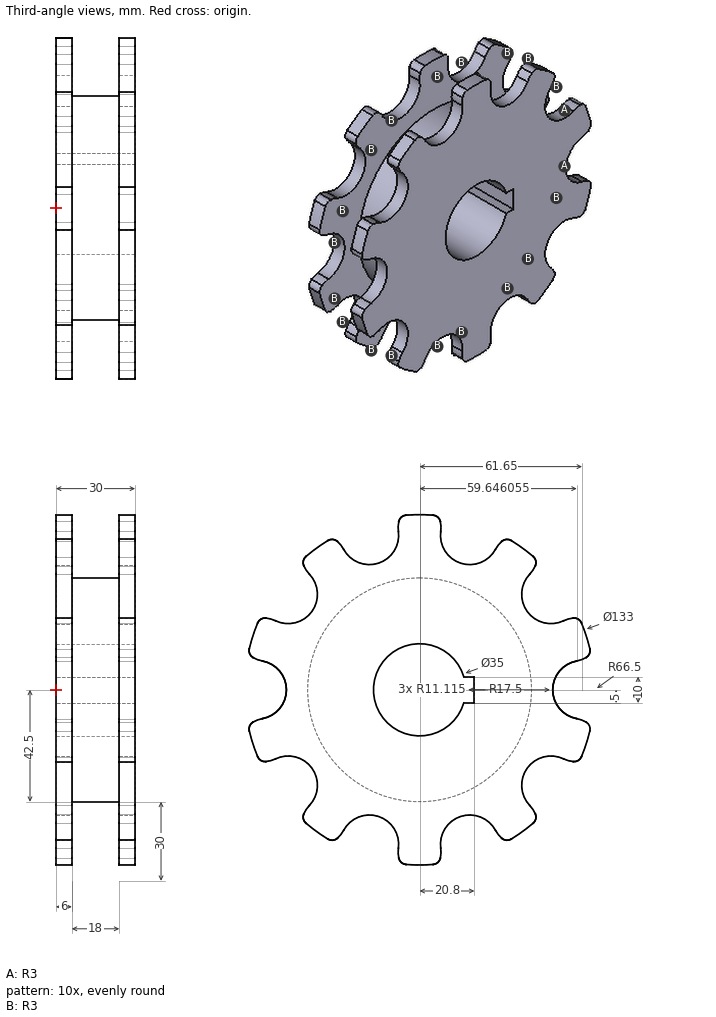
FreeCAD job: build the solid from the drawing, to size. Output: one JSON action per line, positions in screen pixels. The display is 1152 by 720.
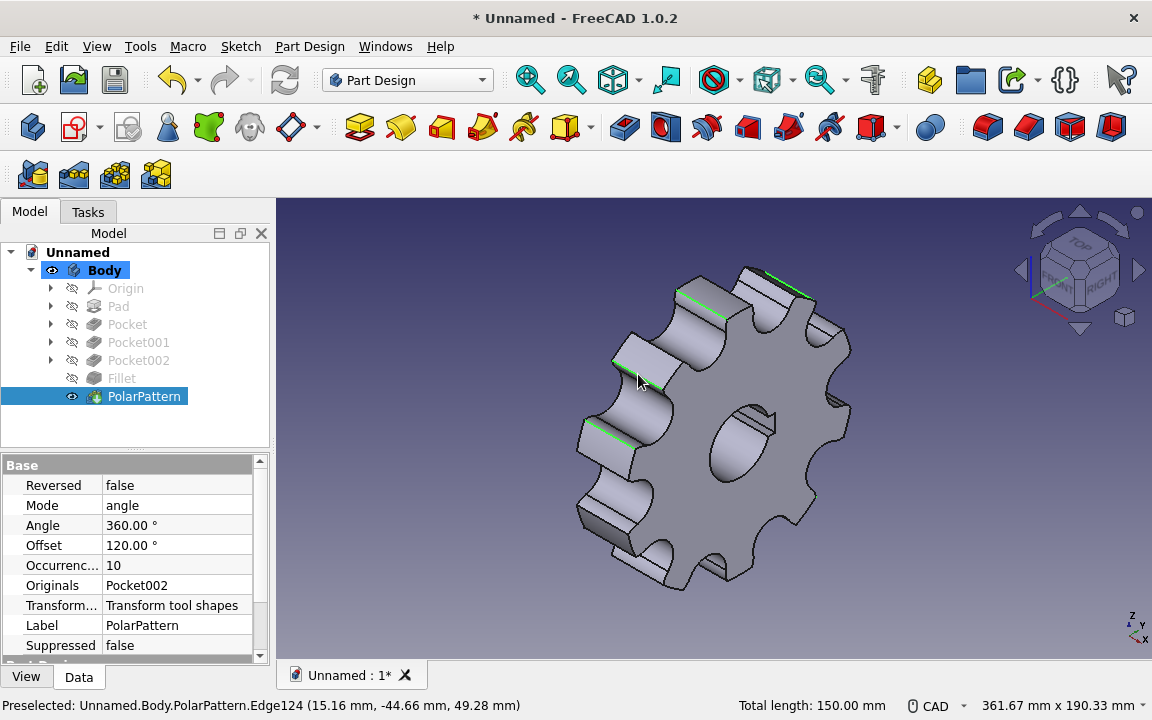
{"action": "left_click", "coordinate": [603, 519], "text": "ctrl"}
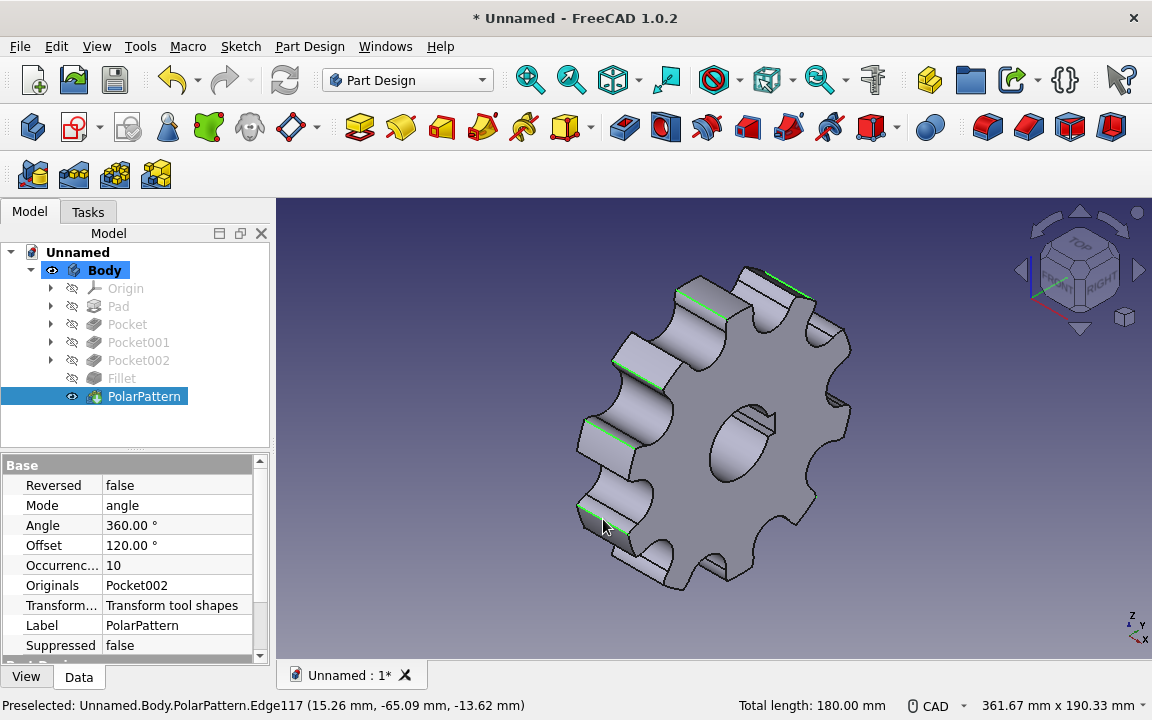
{"action": "key", "text": "2"}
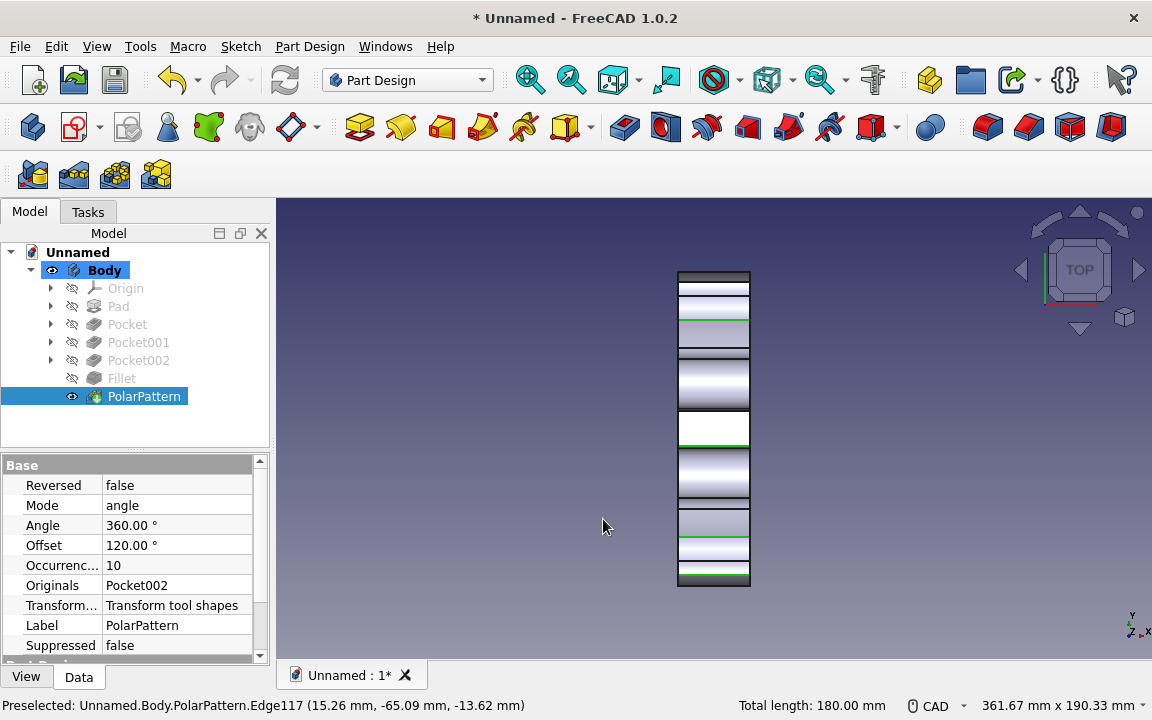
{"action": "left_click", "coordinate": [714, 347], "text": "ctrl"}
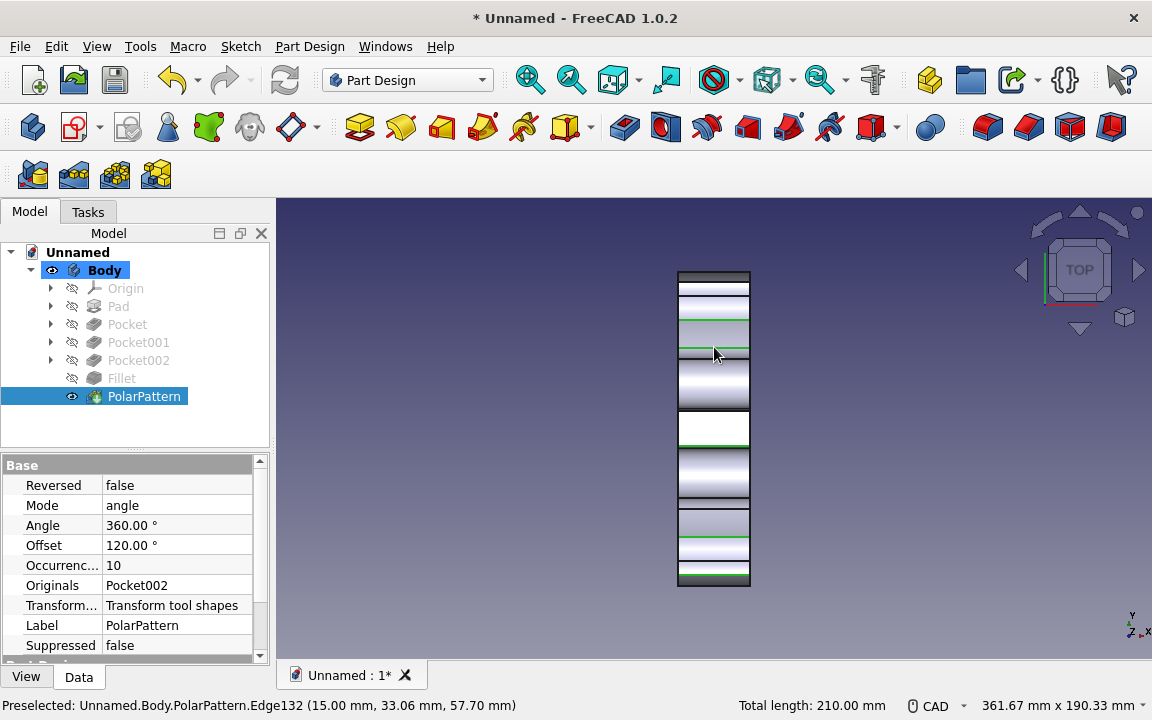
{"action": "left_click", "coordinate": [714, 508], "text": "ctrl"}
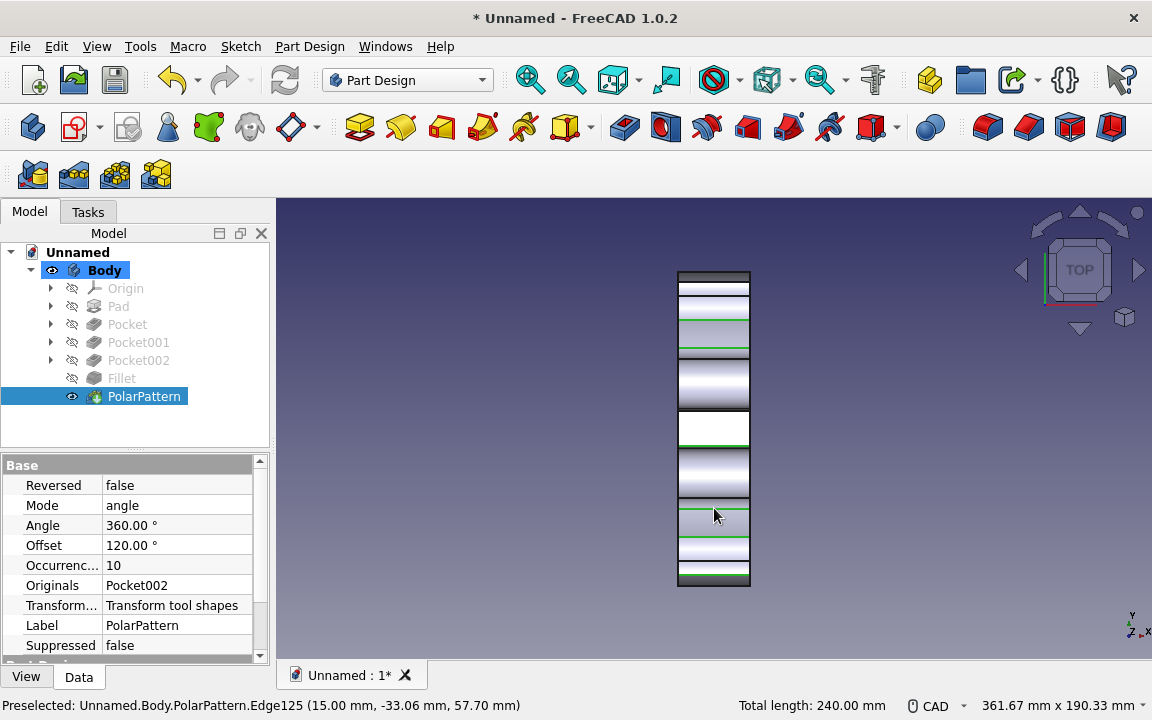
{"action": "key", "text": "1"}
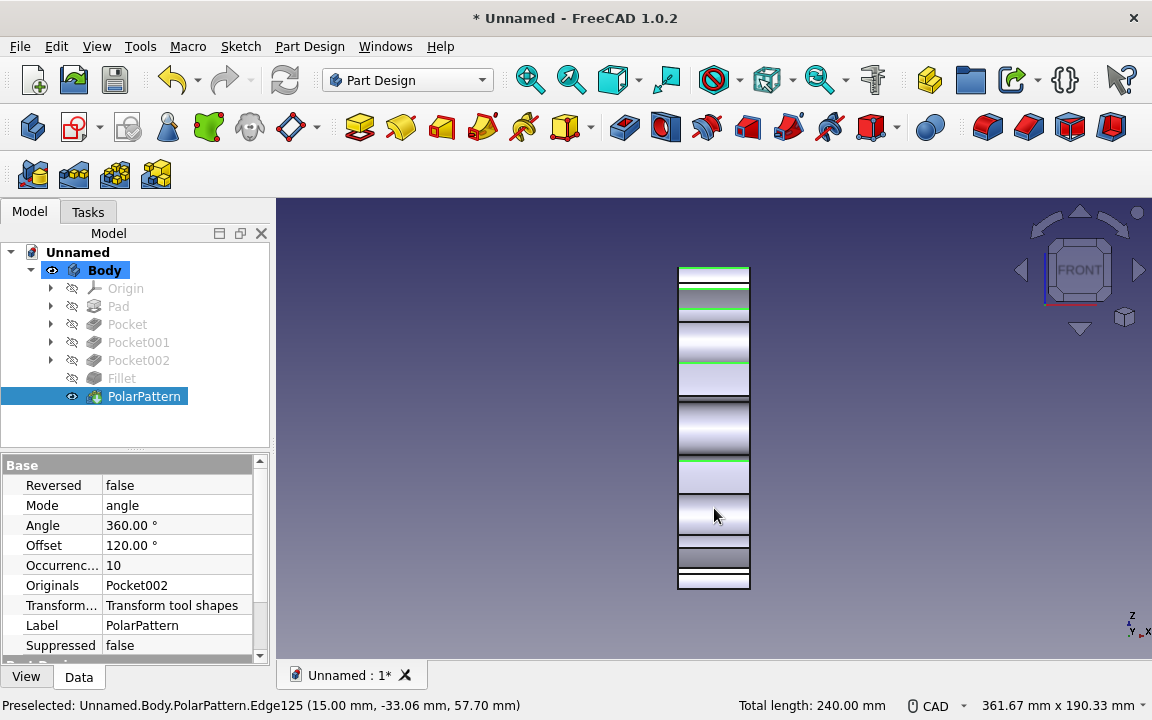
{"action": "left_click", "coordinate": [714, 395], "text": "ctrl"}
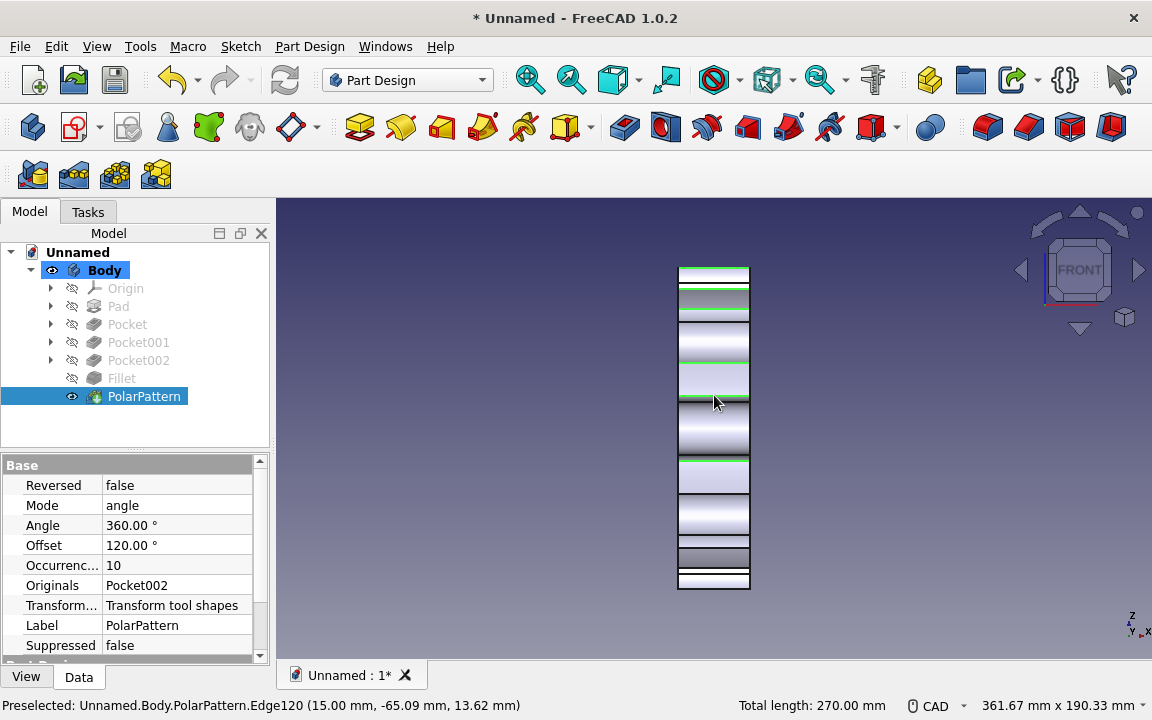
{"action": "left_click", "coordinate": [714, 547], "text": "ctrl"}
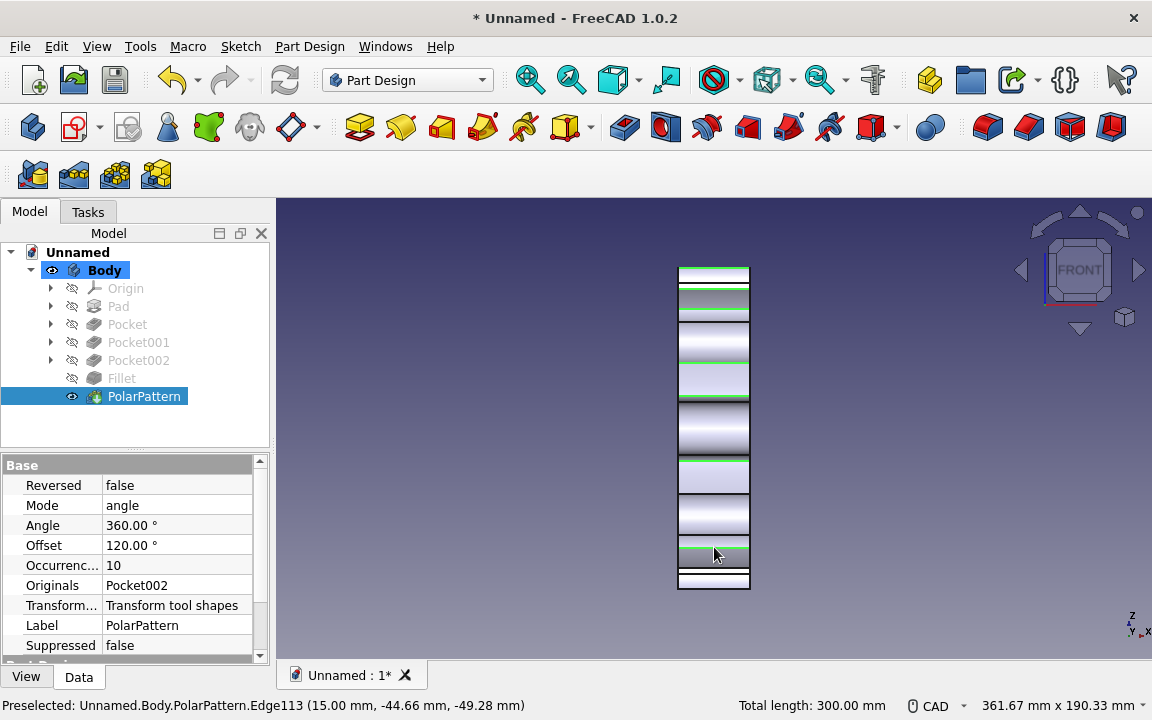
{"action": "key", "text": "3"}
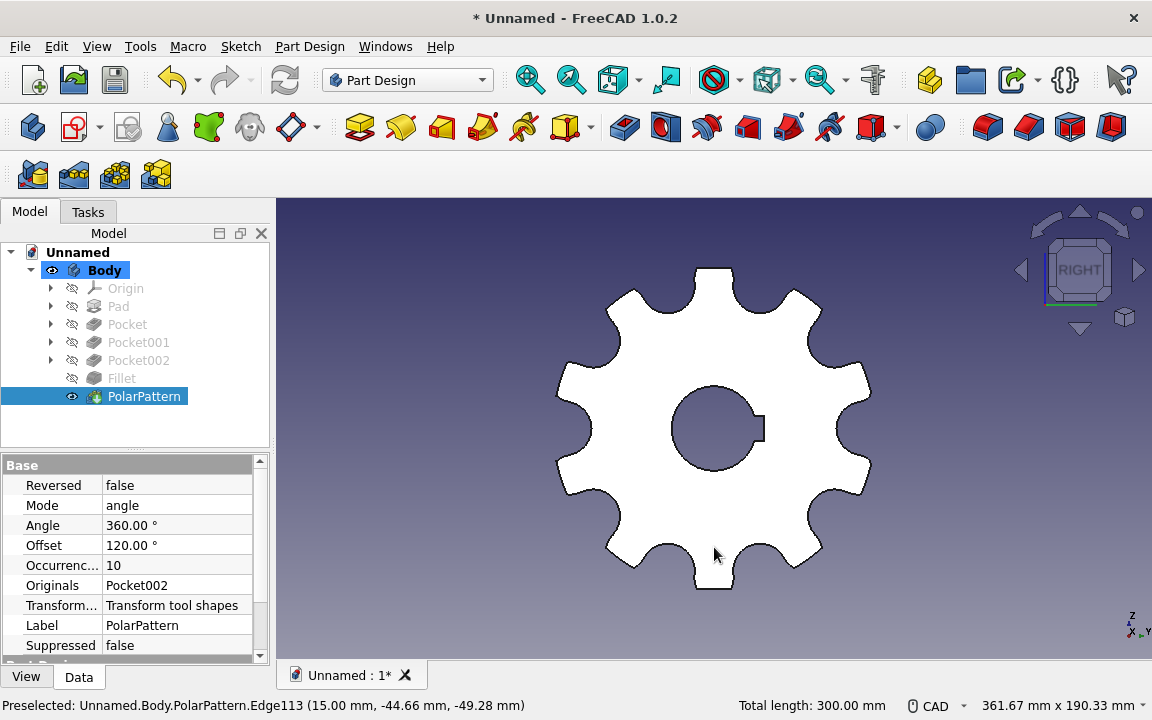
{"action": "key", "text": "5"}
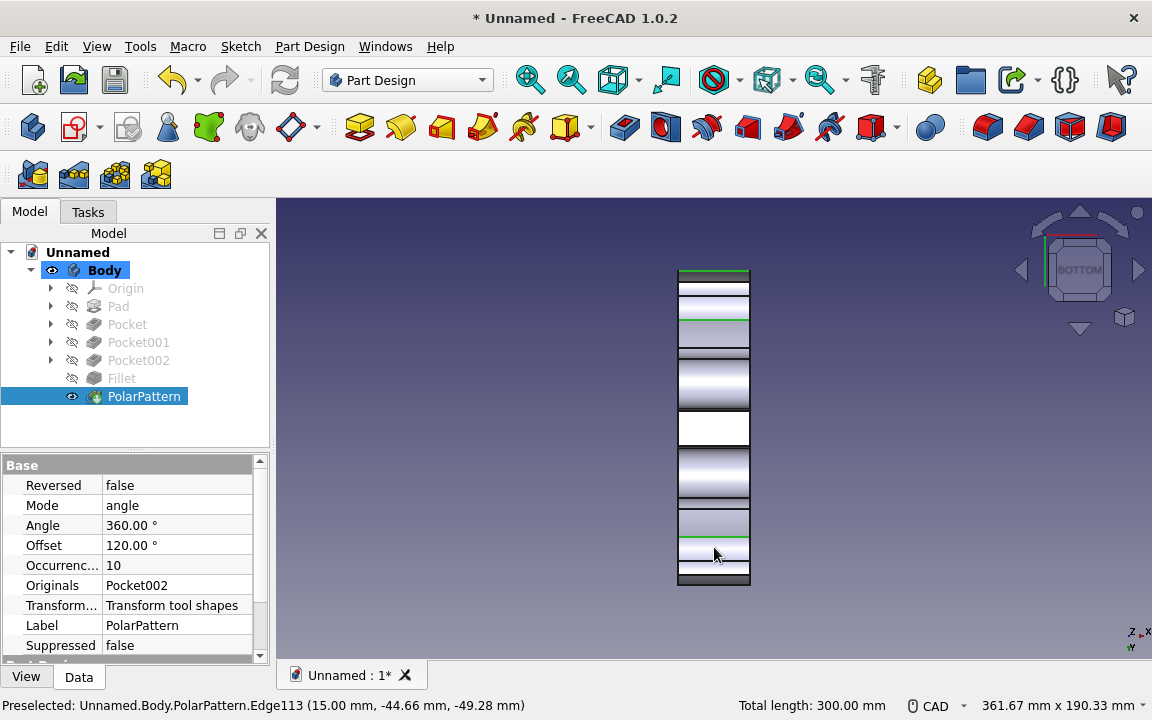
{"action": "left_click", "coordinate": [714, 347], "text": "ctrl"}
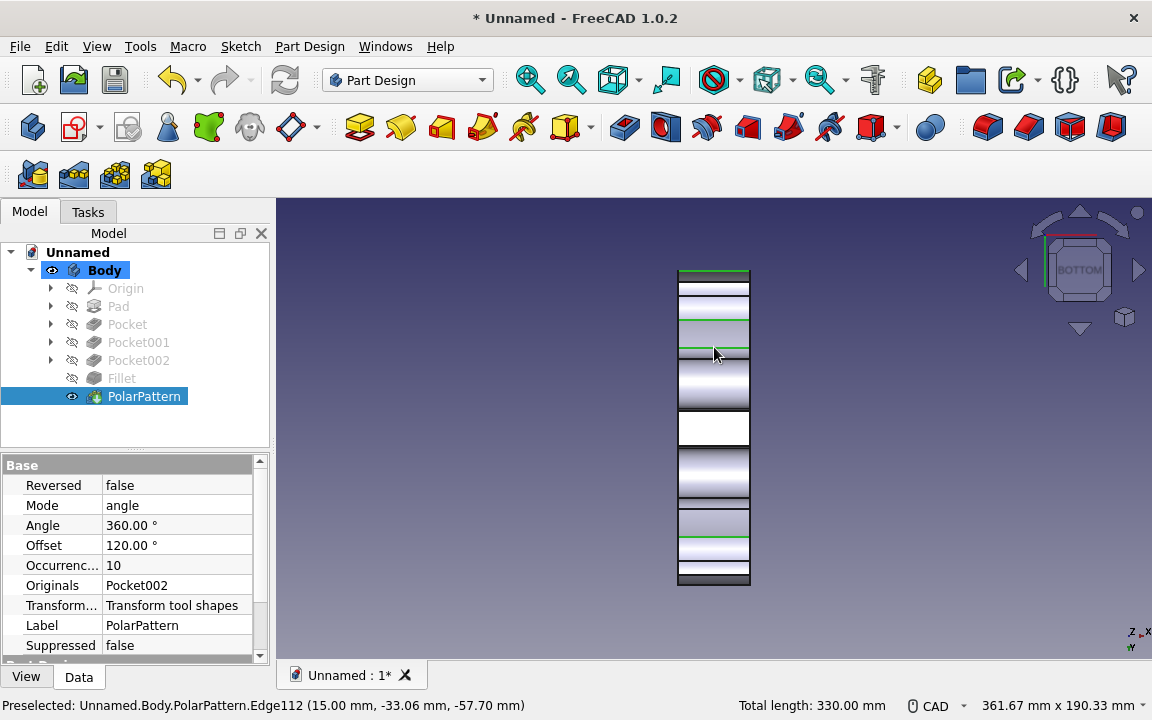
{"action": "left_click", "coordinate": [714, 508], "text": "ctrl"}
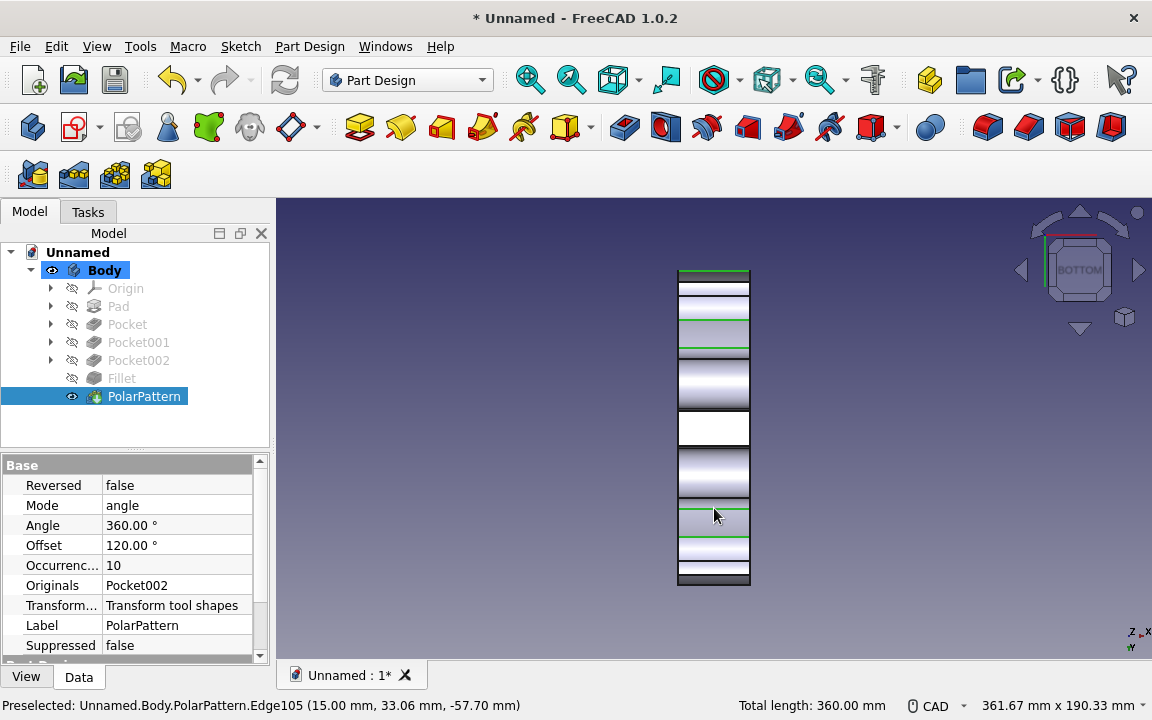
{"action": "key", "text": "4"}